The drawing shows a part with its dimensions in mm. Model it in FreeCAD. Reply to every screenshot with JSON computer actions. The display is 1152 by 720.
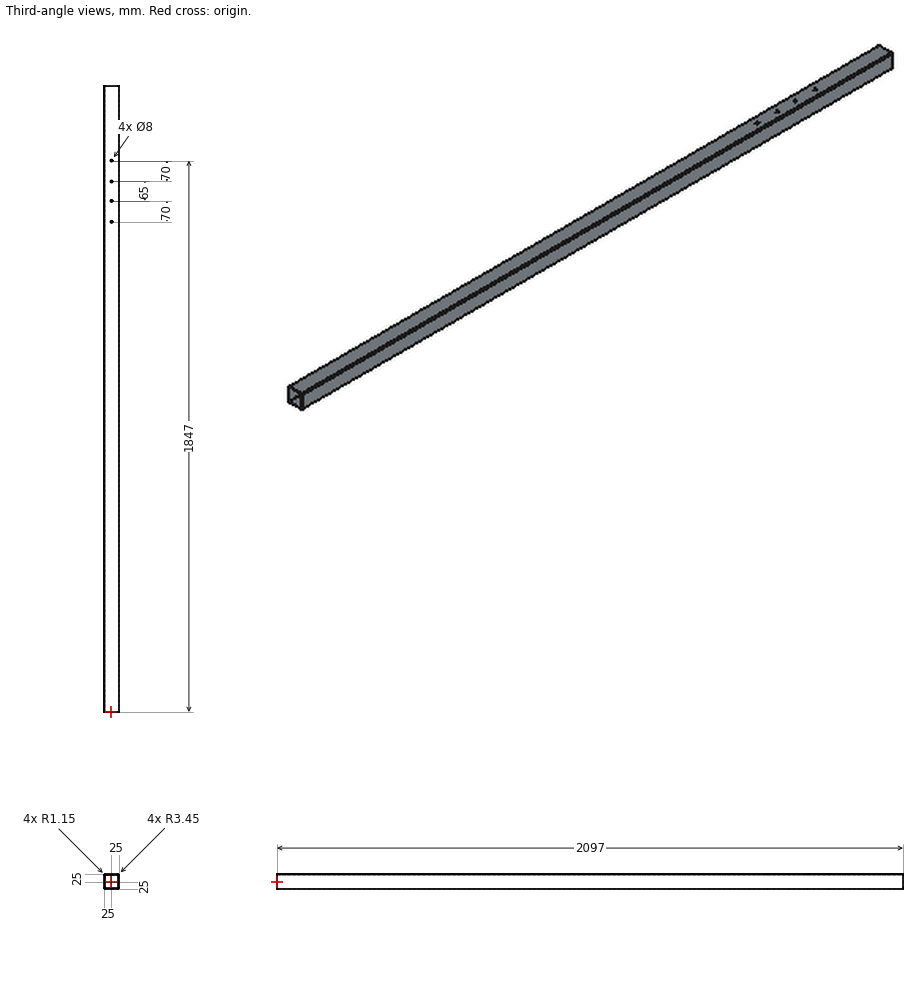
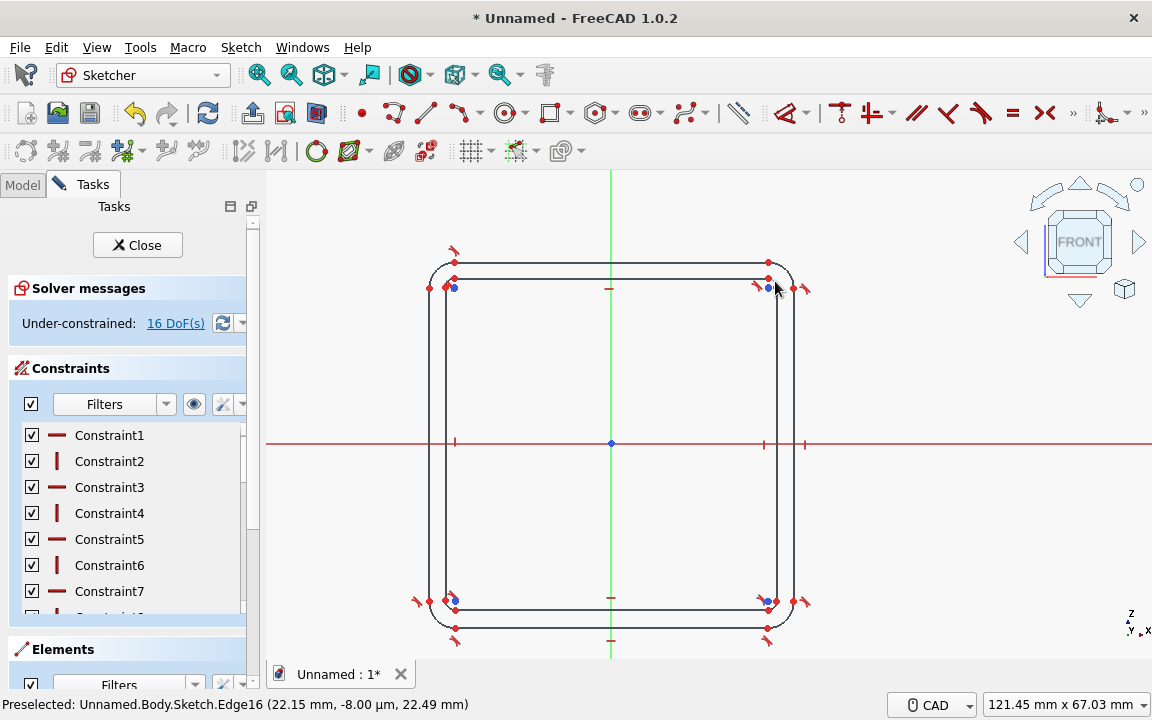
{"action": "scroll", "coordinate": [503, 268], "scroll_direction": "up", "scroll_amount": 2}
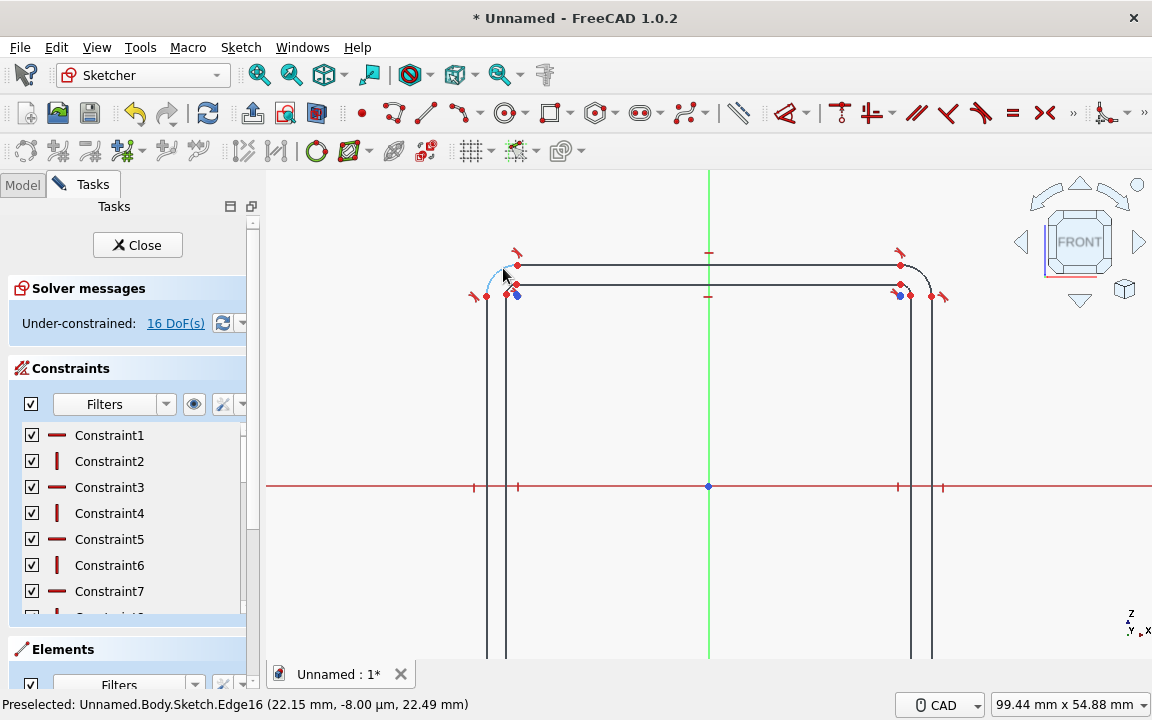
{"action": "left_click", "coordinate": [504, 268]}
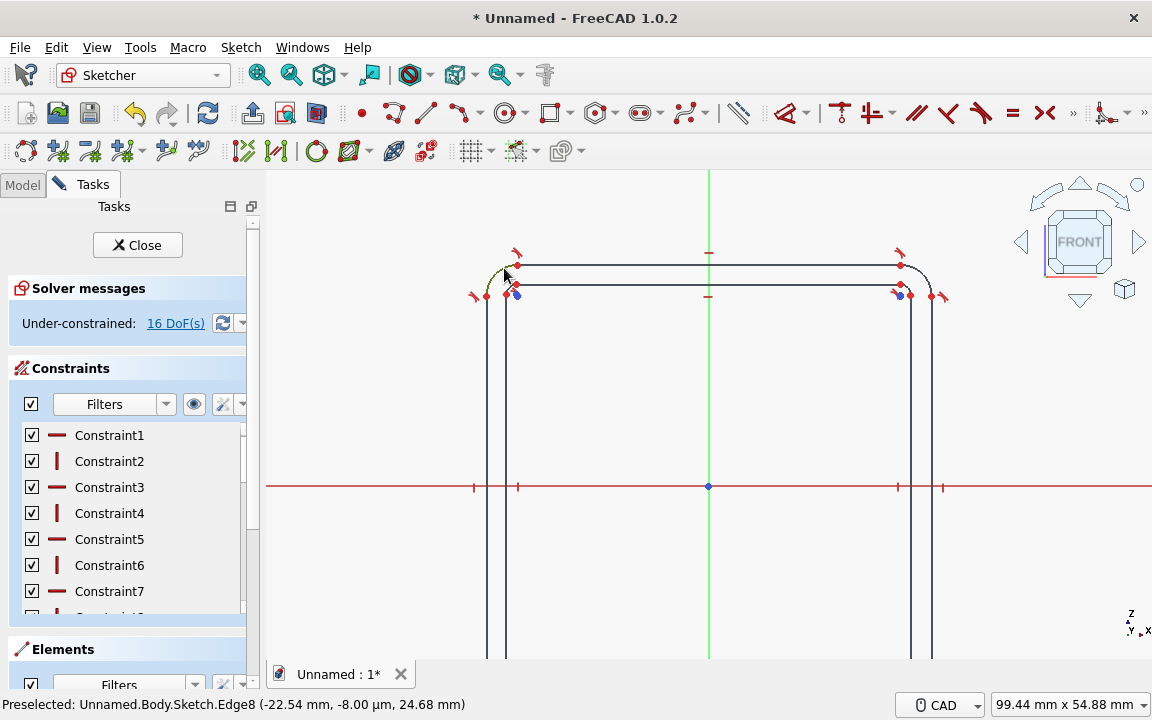
{"action": "scroll", "coordinate": [509, 288], "scroll_direction": "up", "scroll_amount": 3}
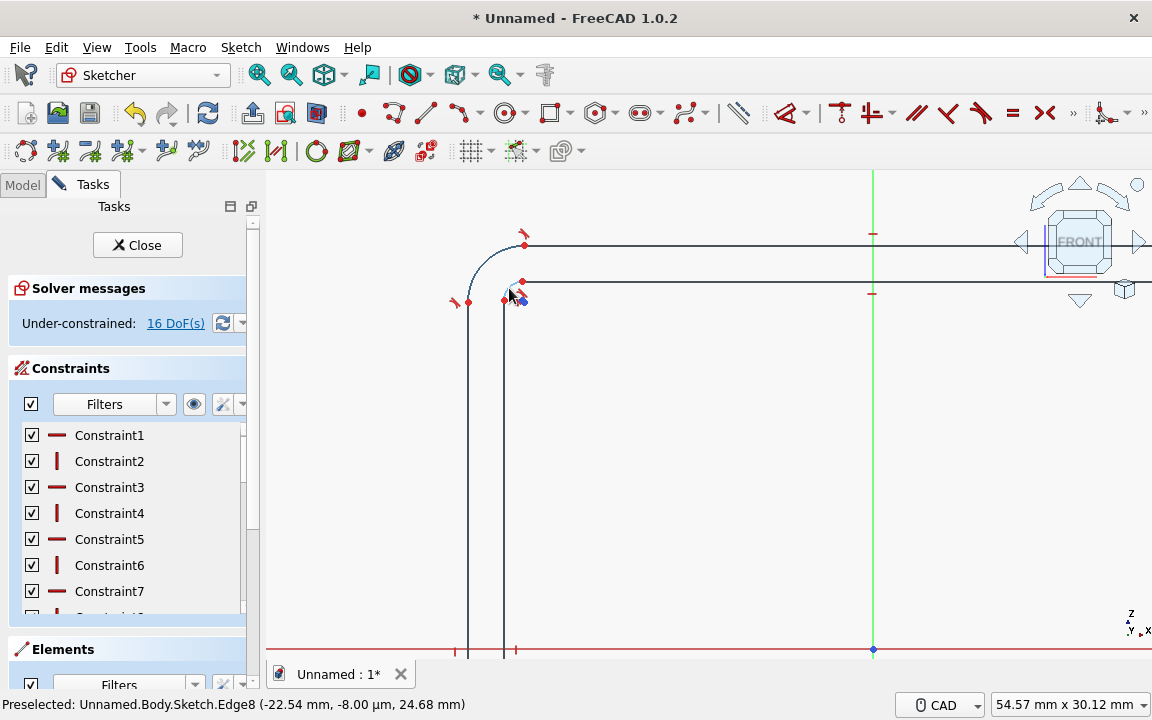
{"action": "left_click", "coordinate": [510, 287]}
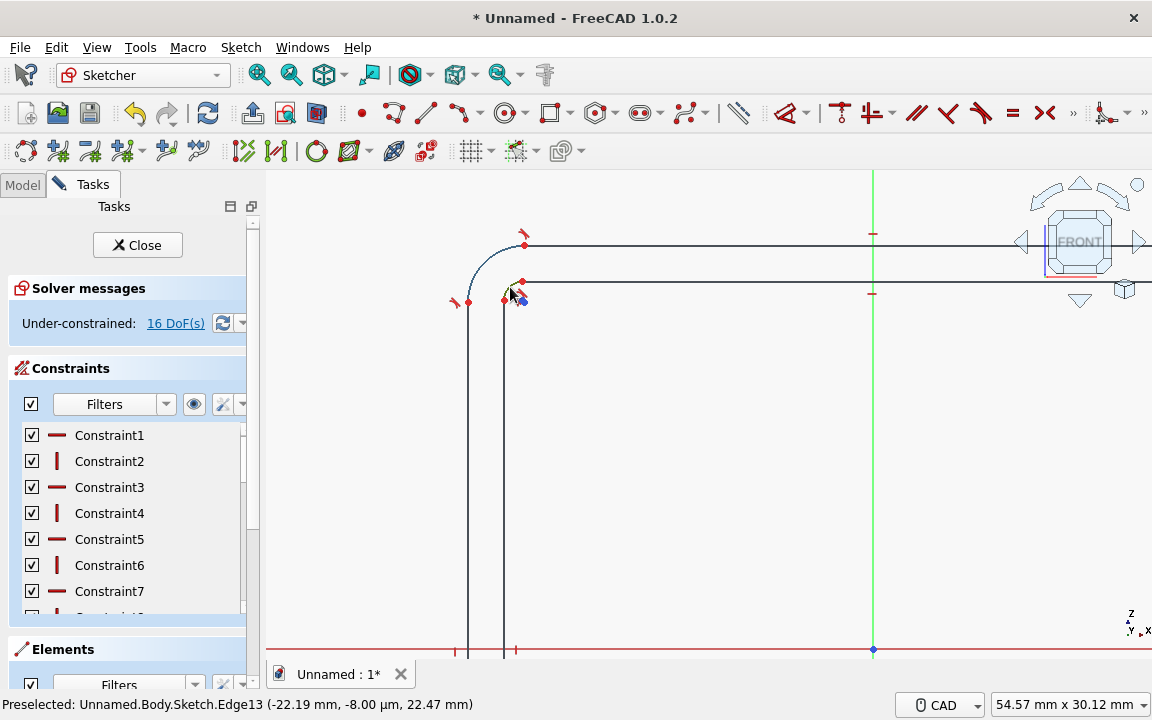
{"action": "left_click", "coordinate": [840, 114]}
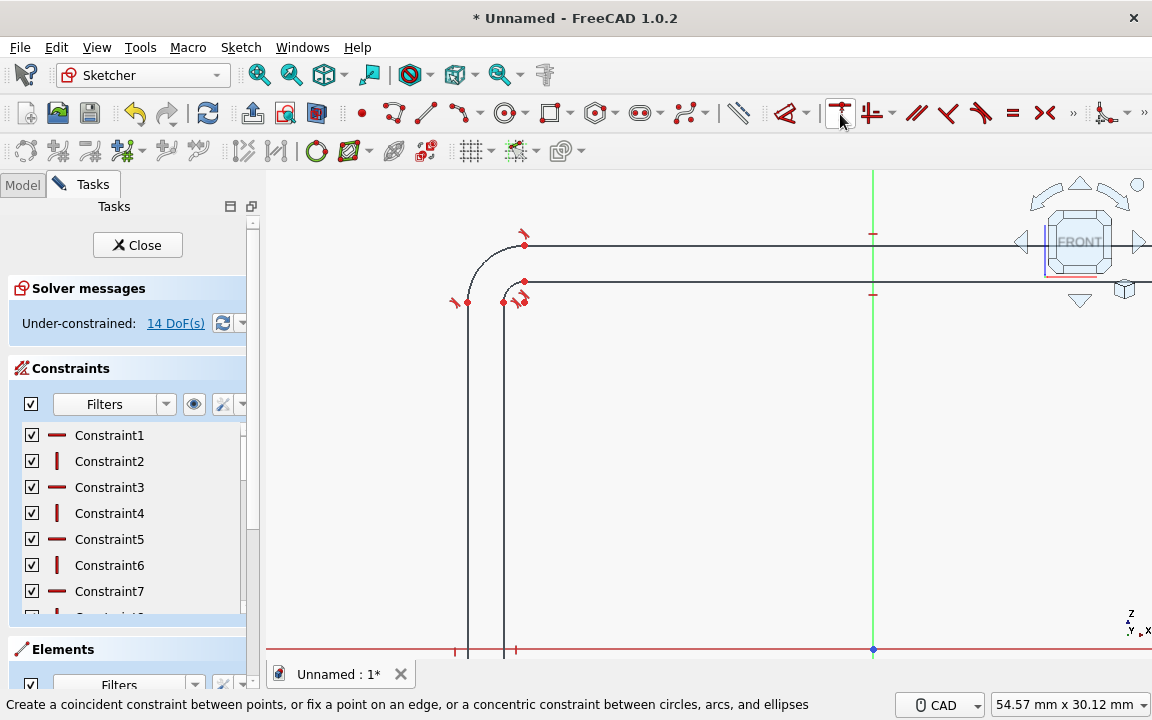
{"action": "scroll", "coordinate": [505, 278], "scroll_direction": "down", "scroll_amount": 5}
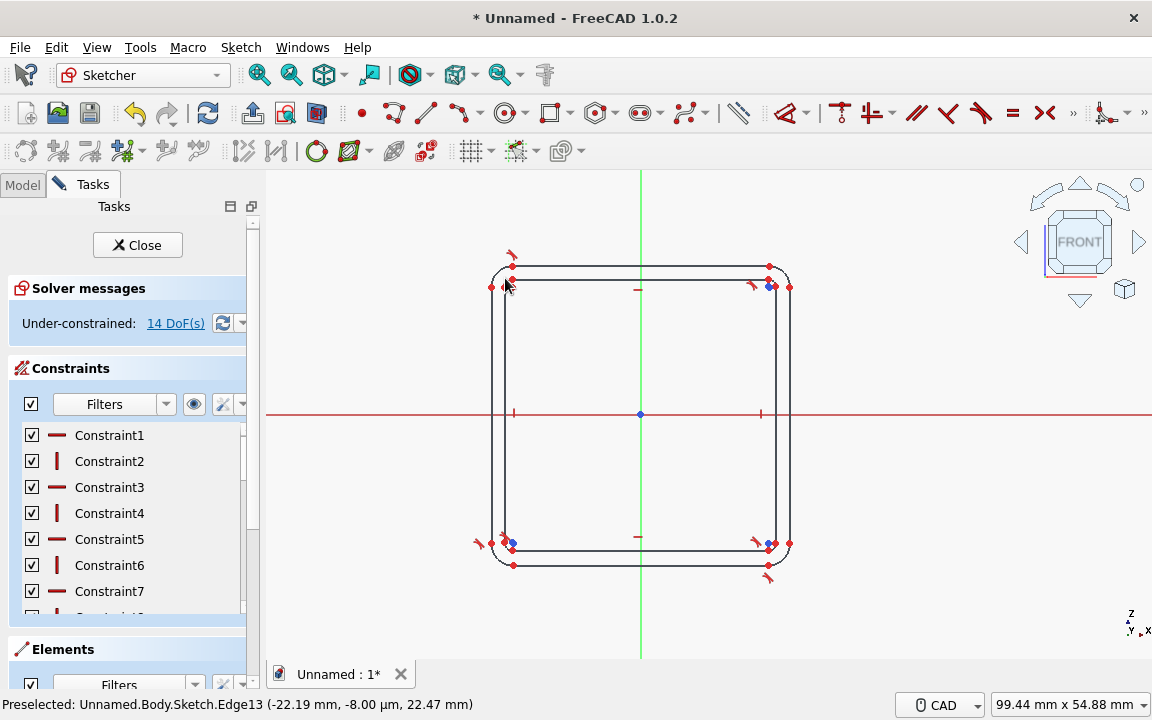
{"action": "scroll", "coordinate": [494, 554], "scroll_direction": "up", "scroll_amount": 2}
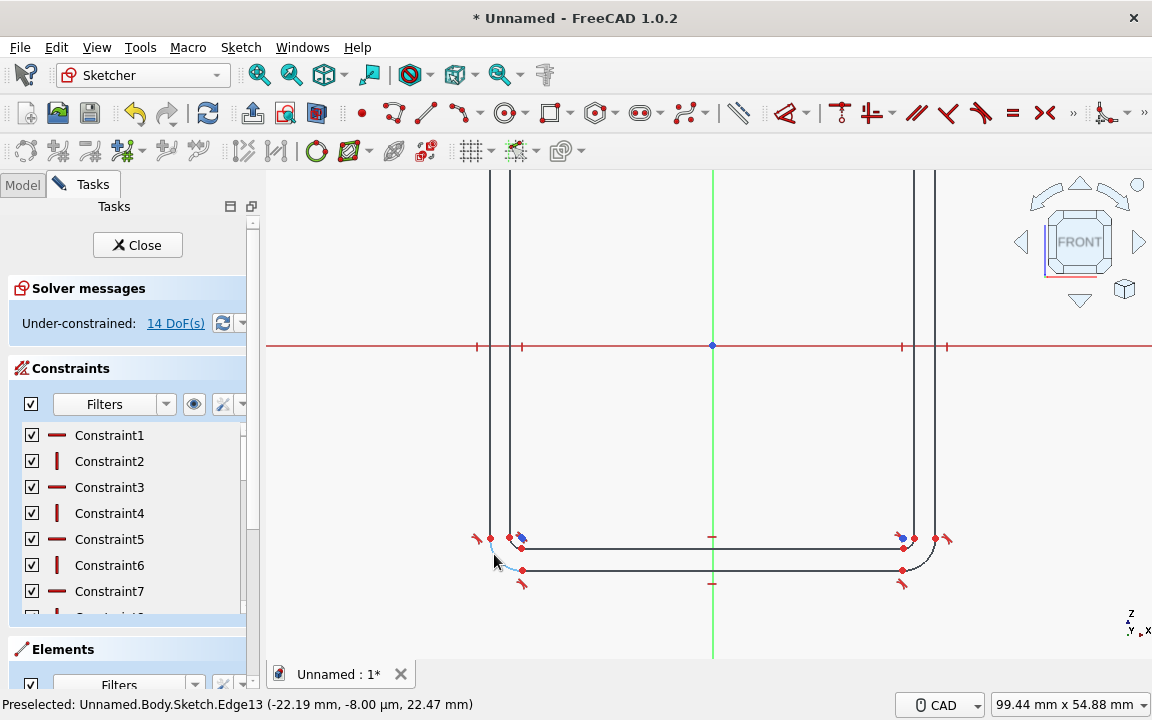
{"action": "left_click", "coordinate": [494, 553]}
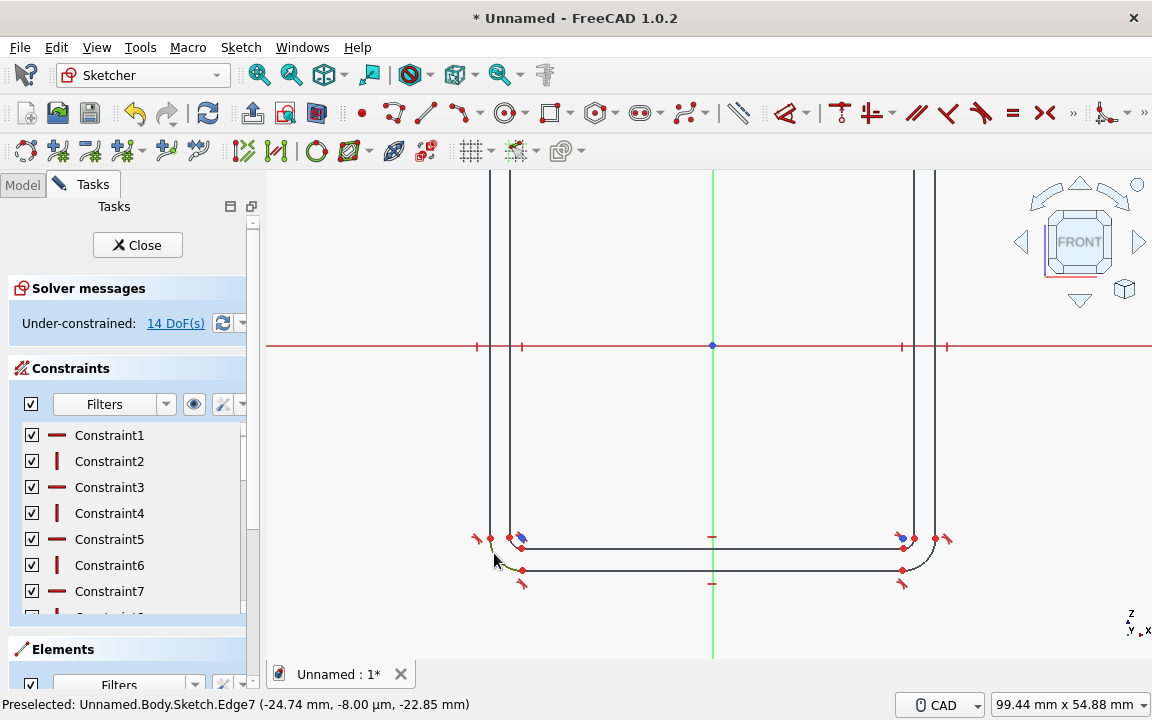
{"action": "scroll", "coordinate": [513, 545], "scroll_direction": "up", "scroll_amount": 3}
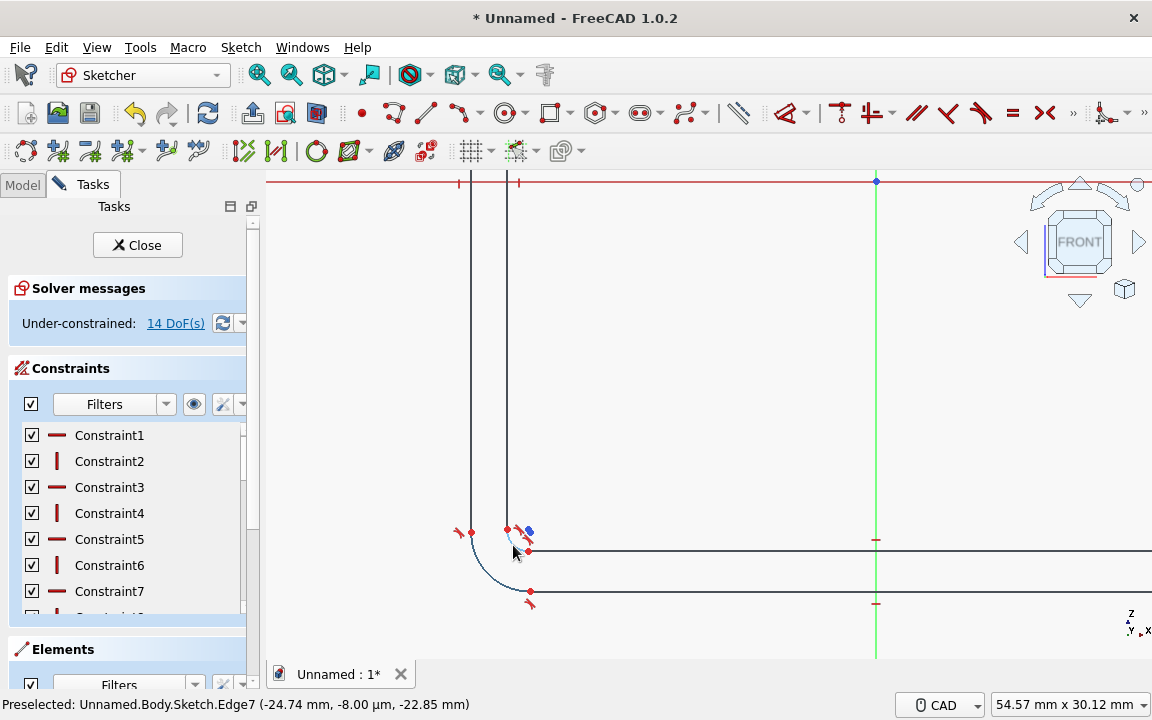
{"action": "left_click", "coordinate": [513, 545]}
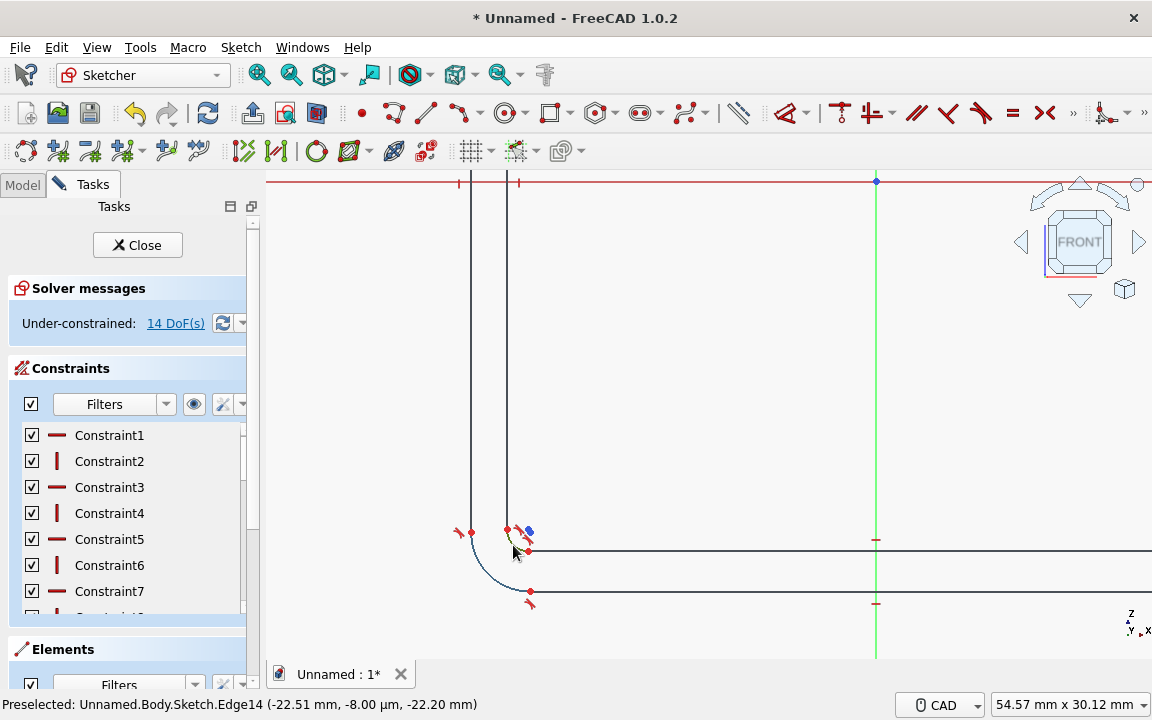
{"action": "left_click", "coordinate": [840, 114]}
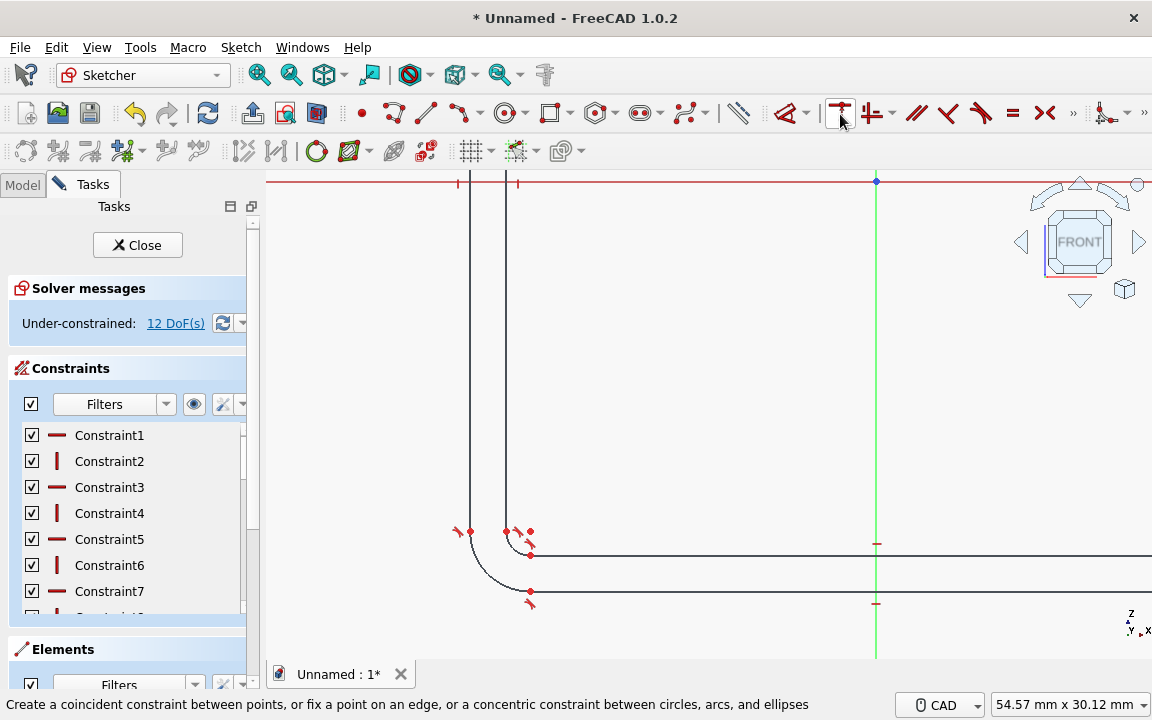
{"action": "scroll", "coordinate": [503, 550], "scroll_direction": "down", "scroll_amount": 5}